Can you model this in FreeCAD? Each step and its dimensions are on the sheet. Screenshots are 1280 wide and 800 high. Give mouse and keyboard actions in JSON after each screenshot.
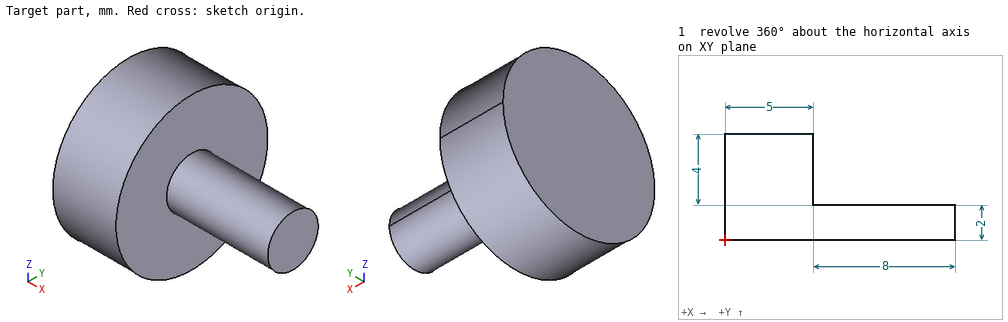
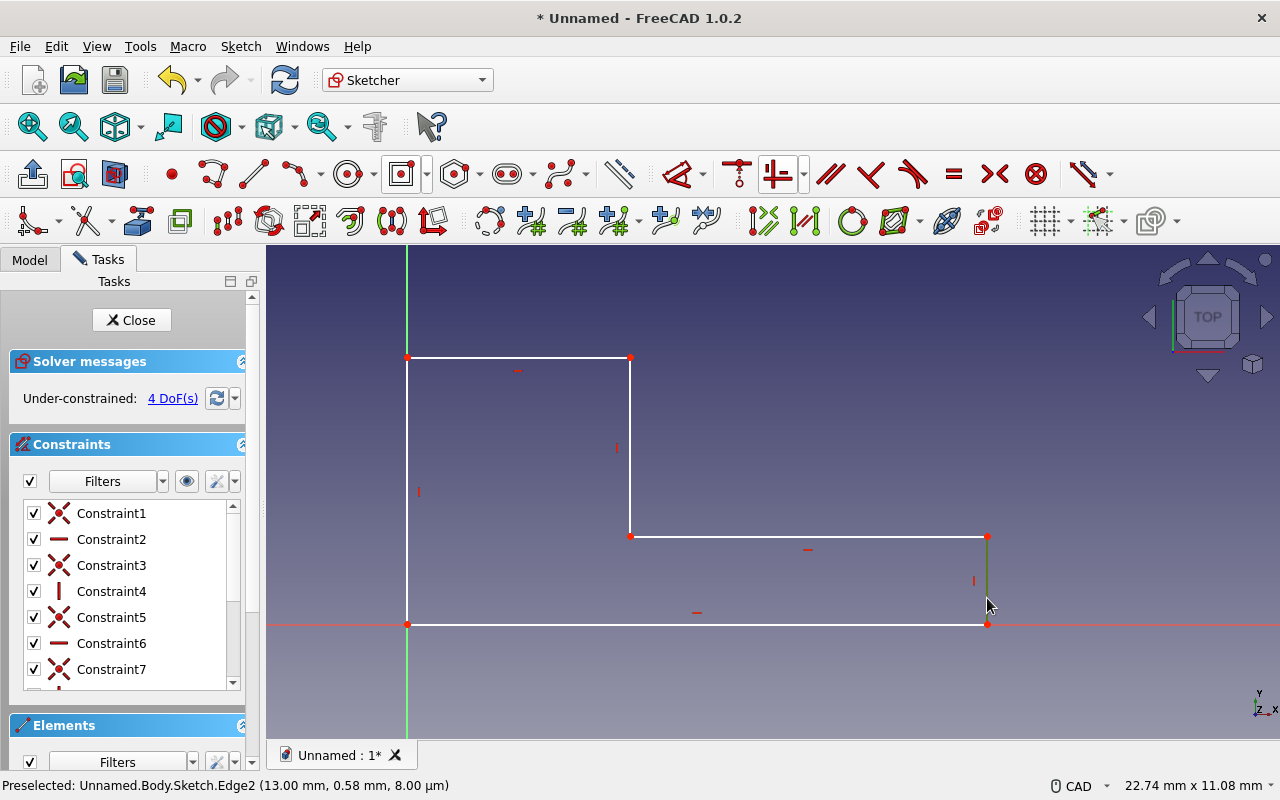
{"action": "key", "text": "i"}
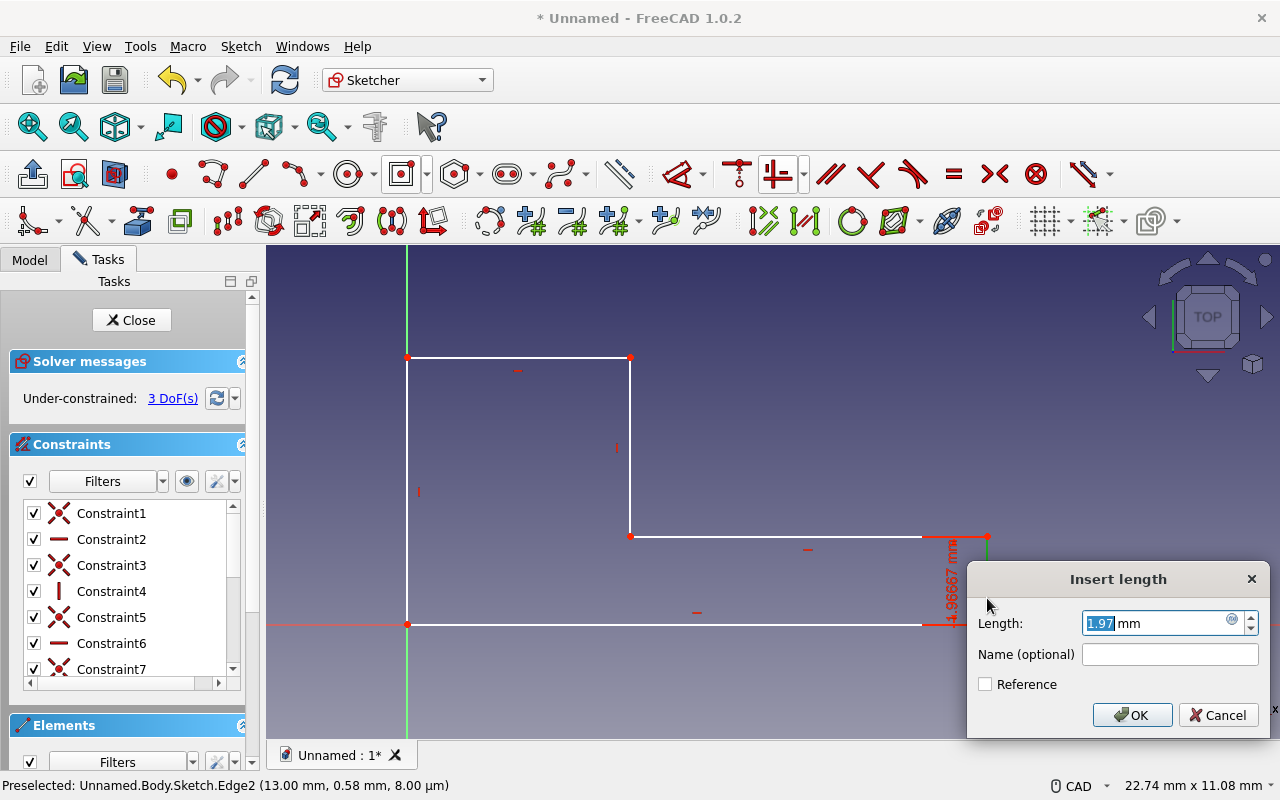
{"action": "type", "text": "2"}
{"action": "key", "text": "Return"}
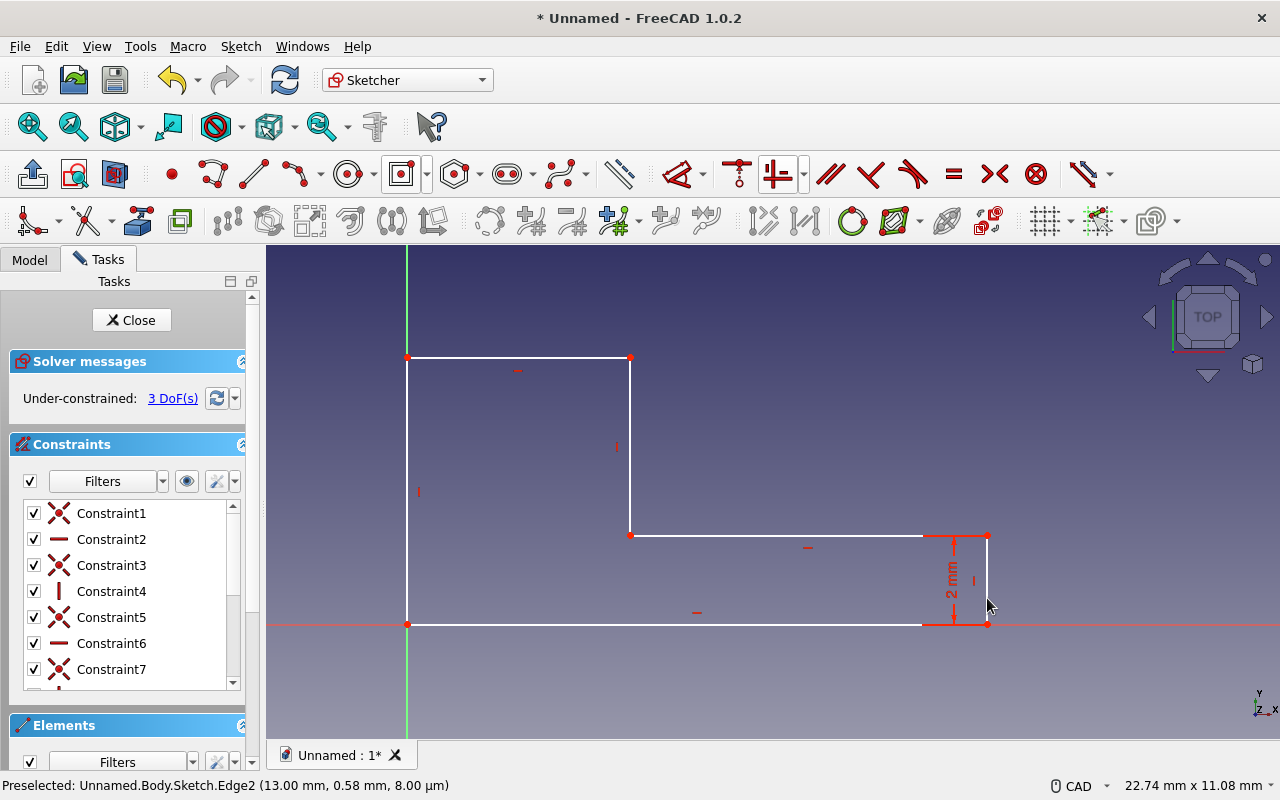
{"action": "left_click", "coordinate": [880, 536]}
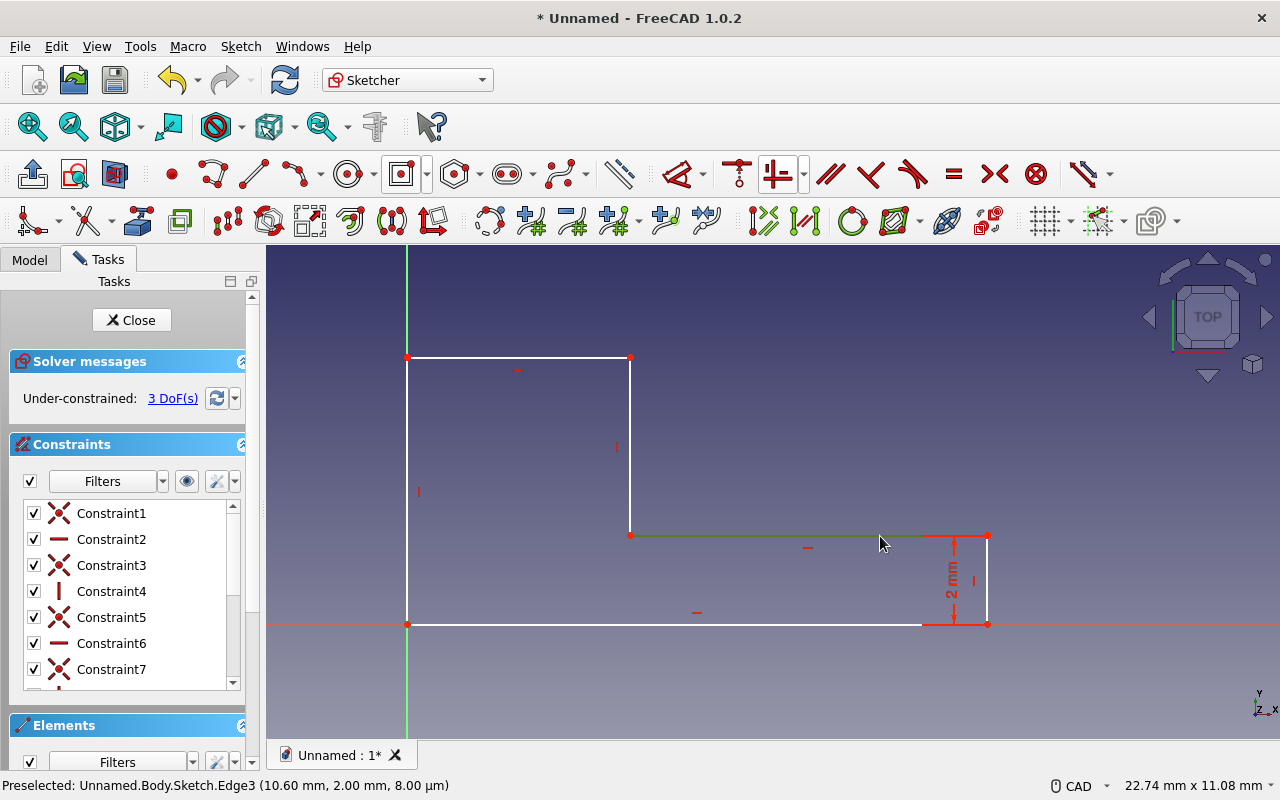
{"action": "key", "text": "l"}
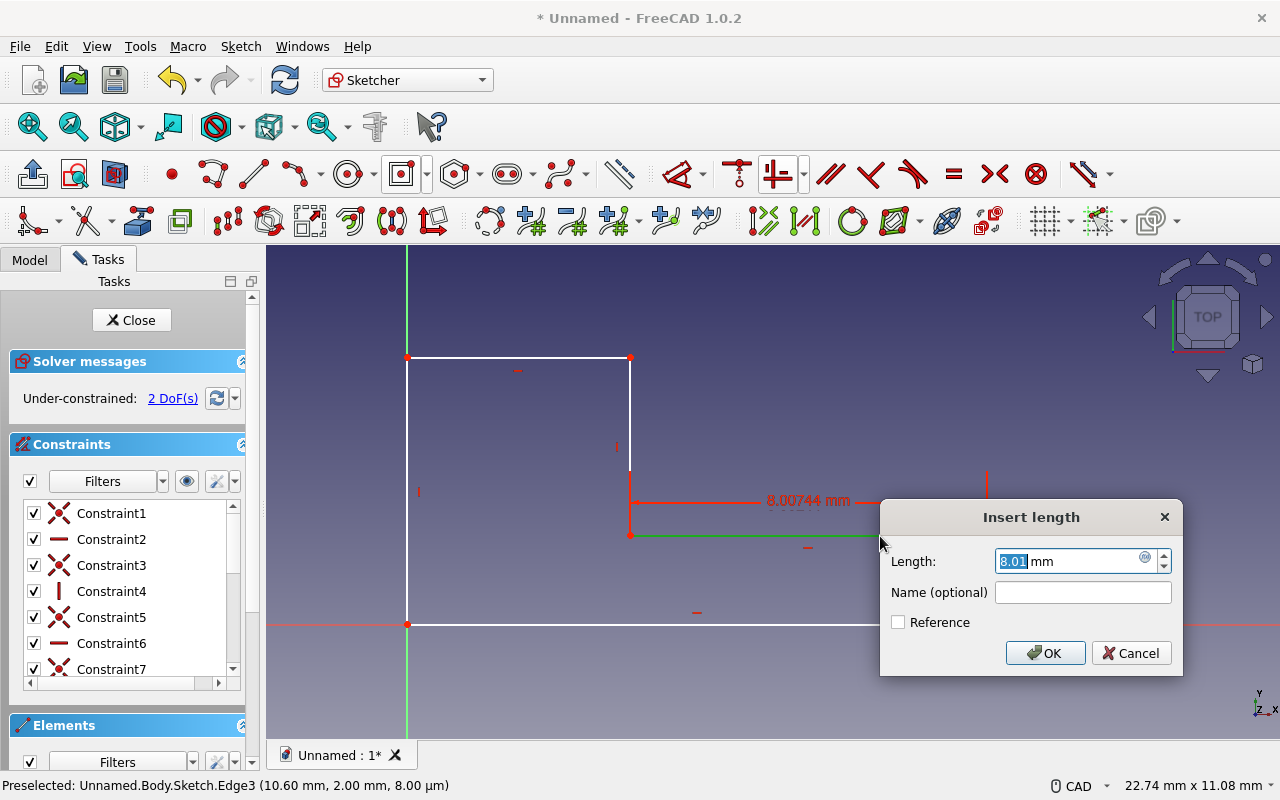
{"action": "type", "text": "8"}
{"action": "key", "text": "Return"}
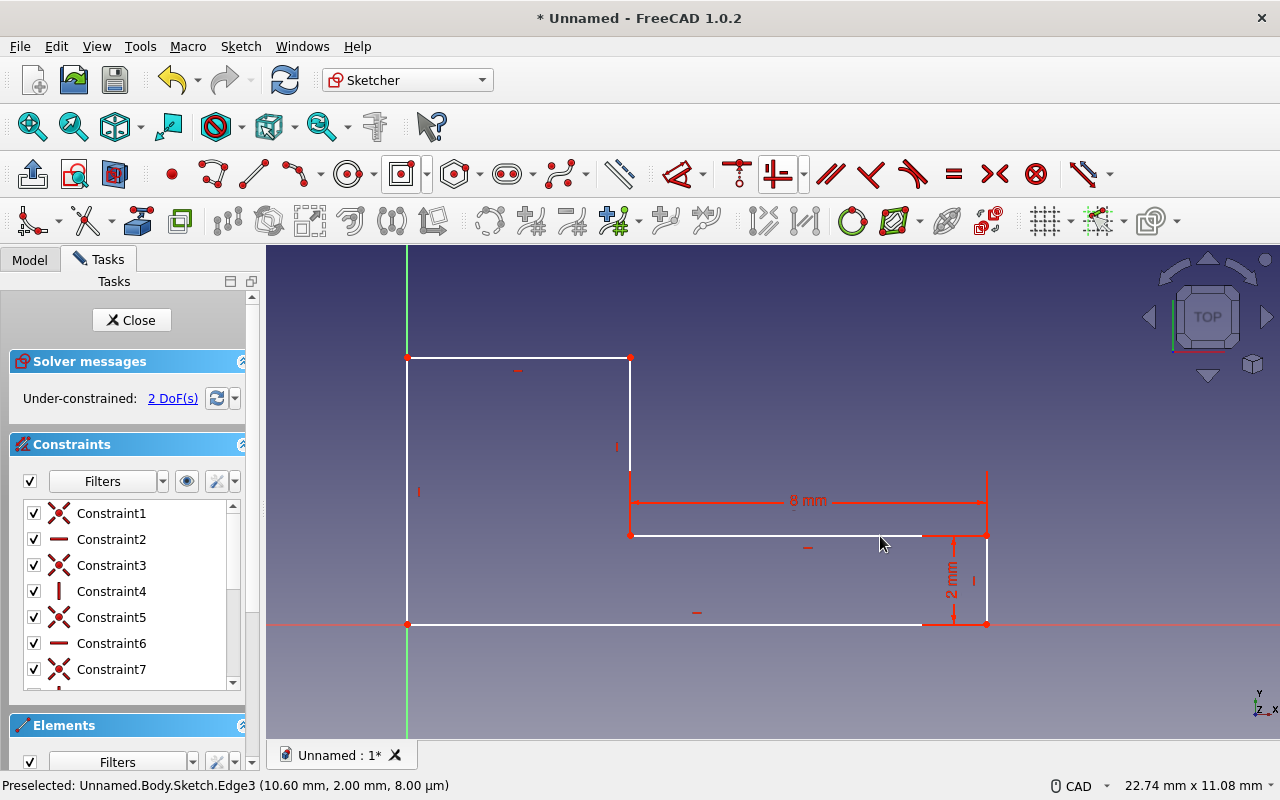
{"action": "left_click", "coordinate": [630, 482]}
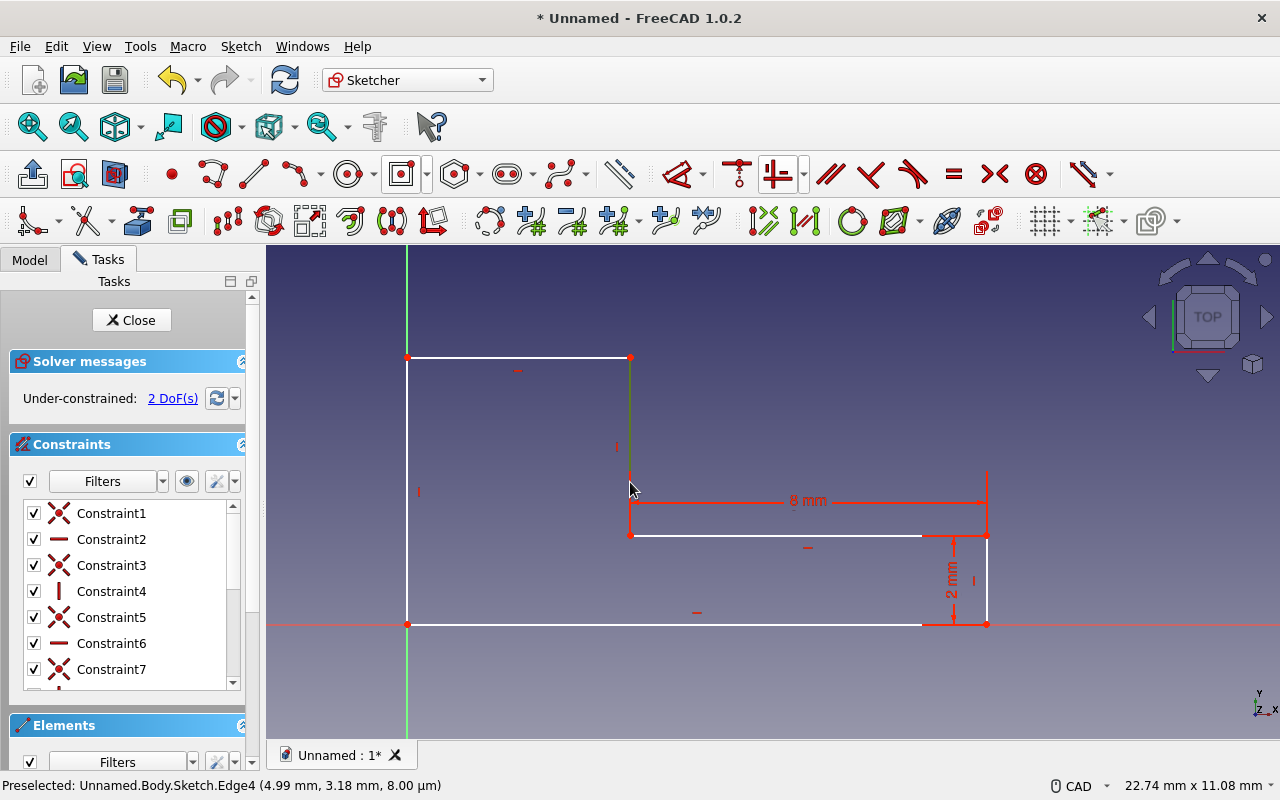
{"action": "key", "text": "i"}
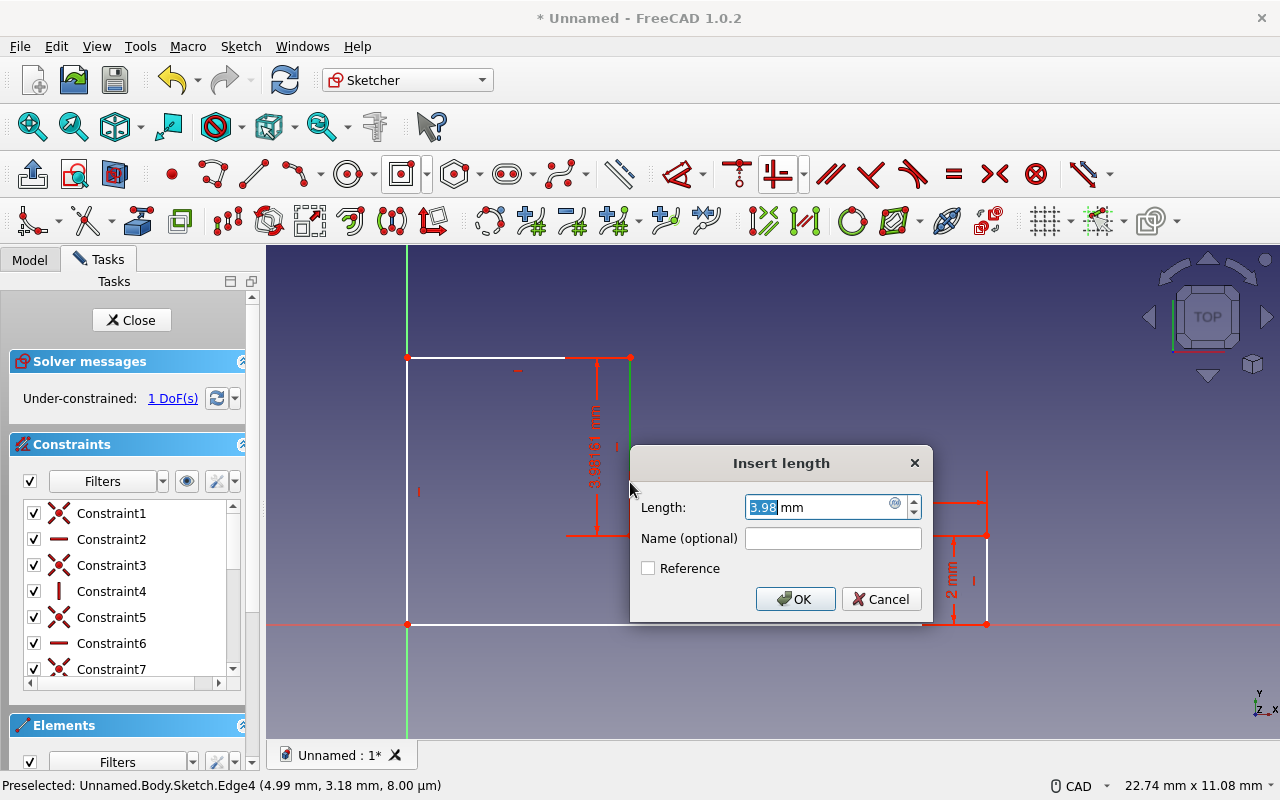
{"action": "type", "text": "4"}
{"action": "key", "text": "Return"}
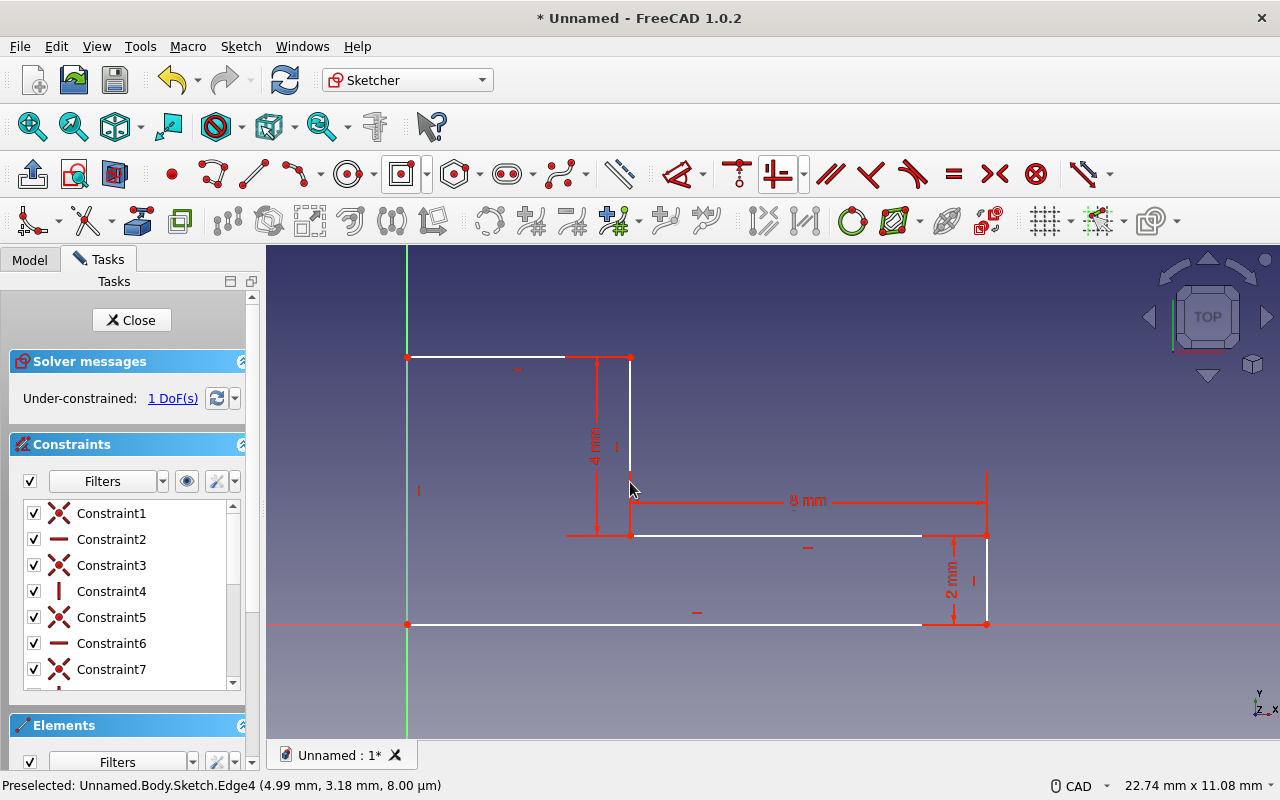
{"action": "left_click", "coordinate": [563, 357]}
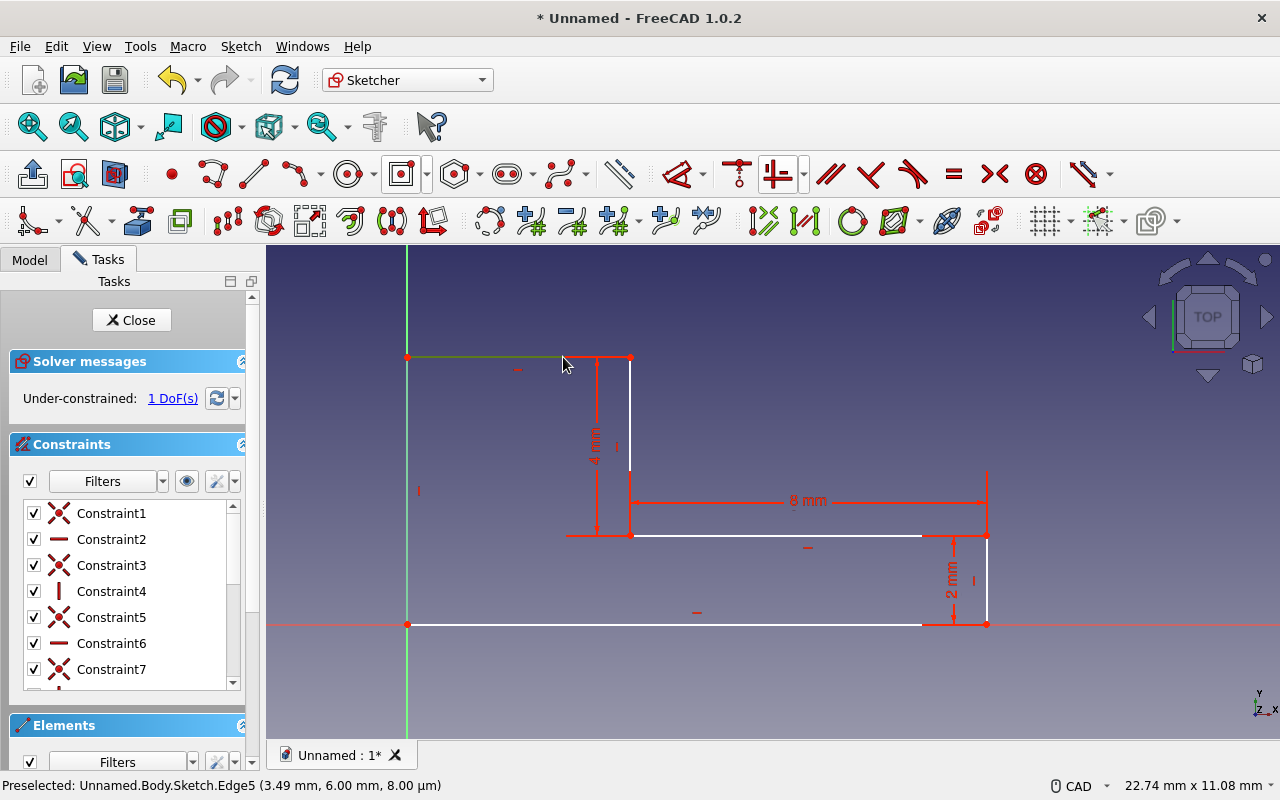
{"action": "key", "text": "l"}